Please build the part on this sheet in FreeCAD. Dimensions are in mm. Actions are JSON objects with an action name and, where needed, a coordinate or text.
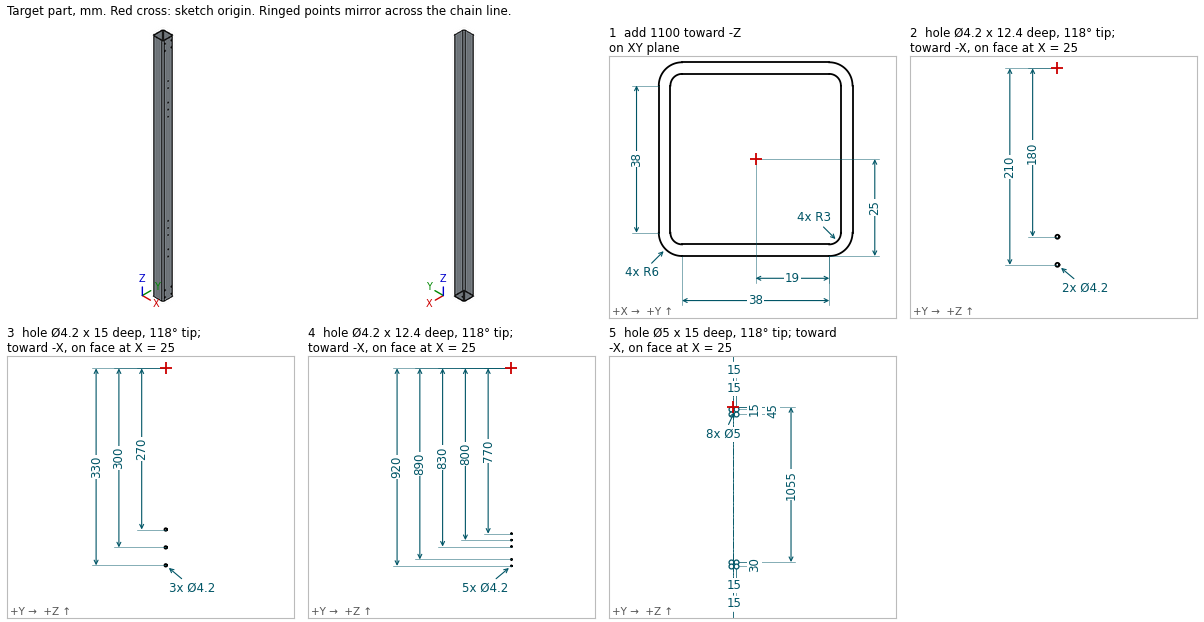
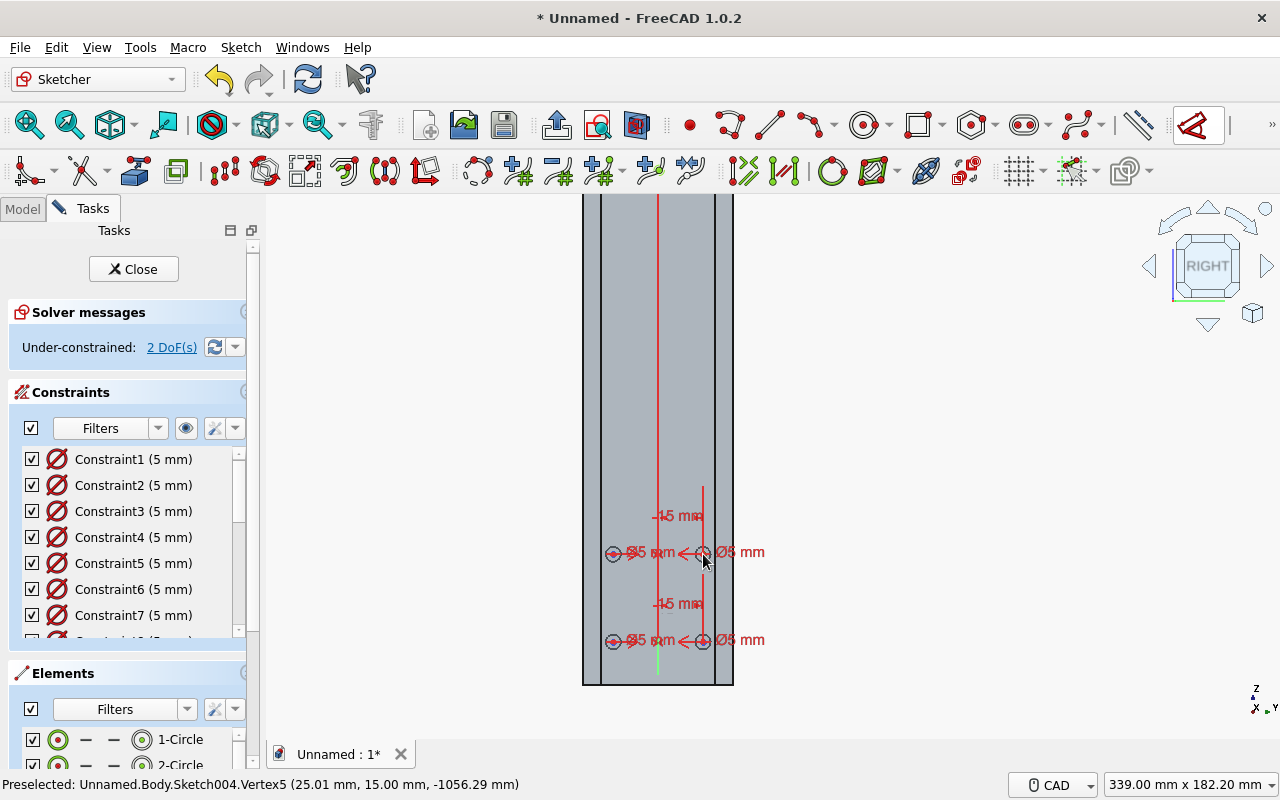
{"action": "left_click", "coordinate": [703, 642]}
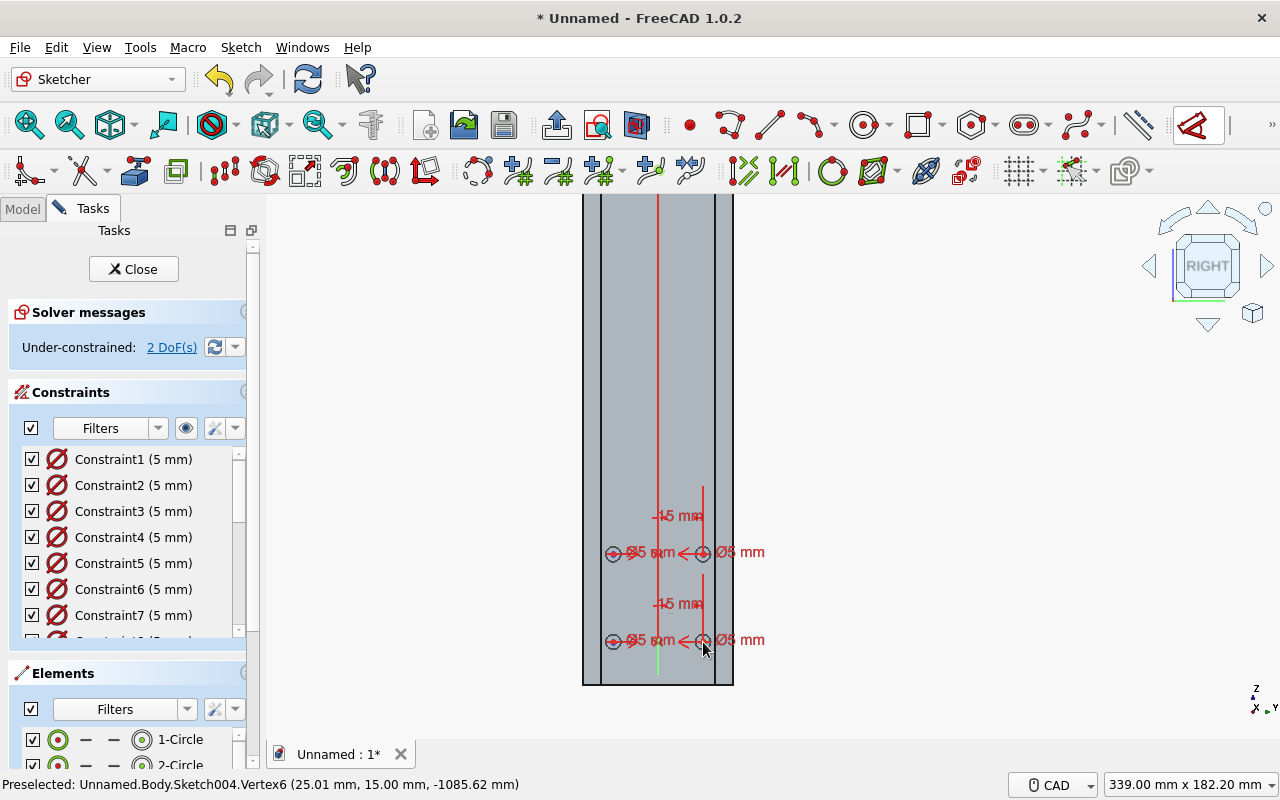
{"action": "left_click", "coordinate": [1218, 126]}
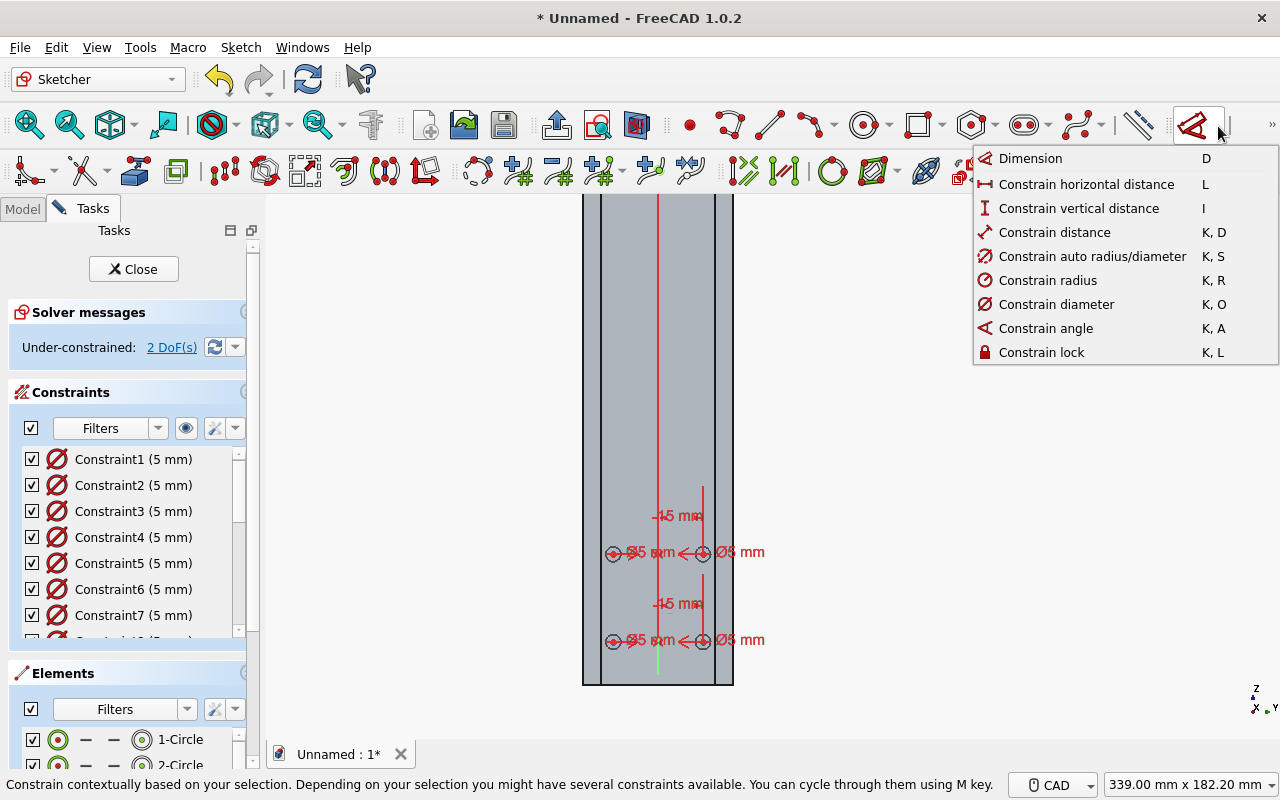
{"action": "left_click", "coordinate": [1126, 208]}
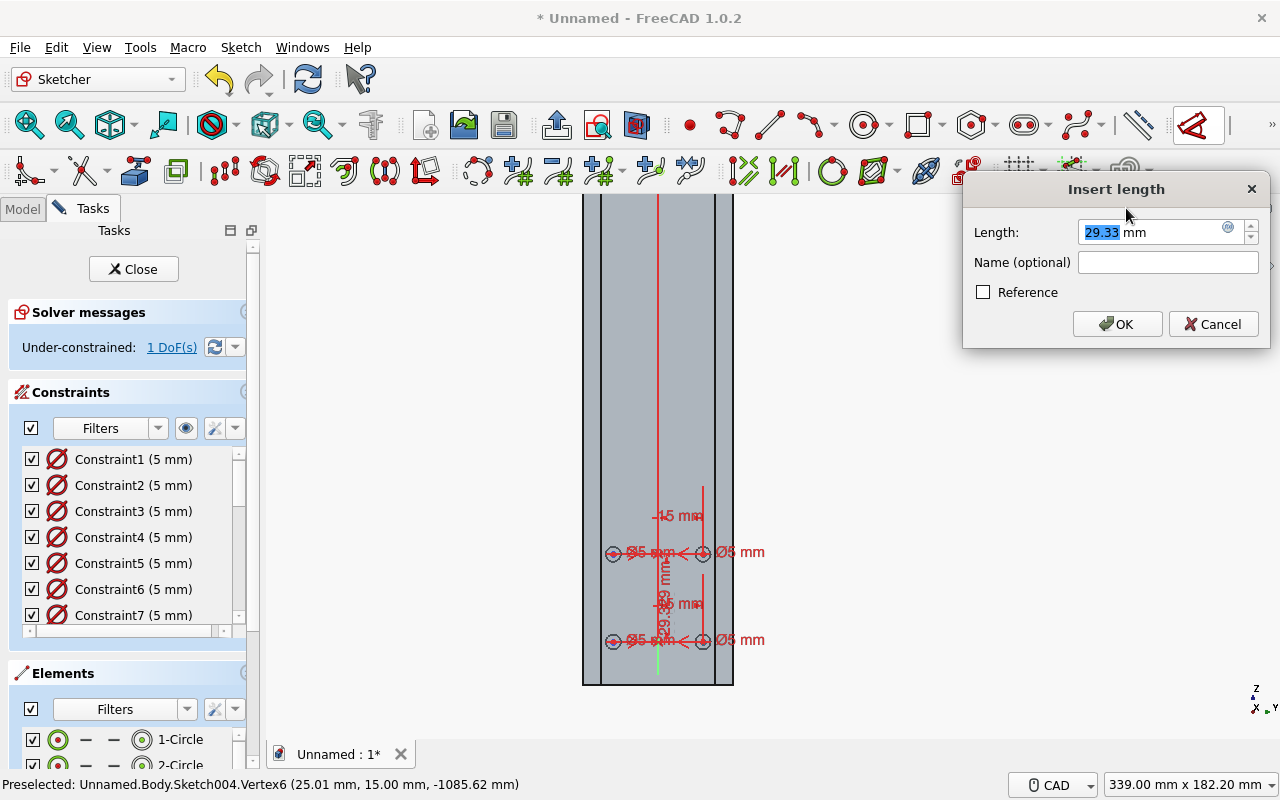
{"action": "type", "text": "30"}
{"action": "key", "text": "Return"}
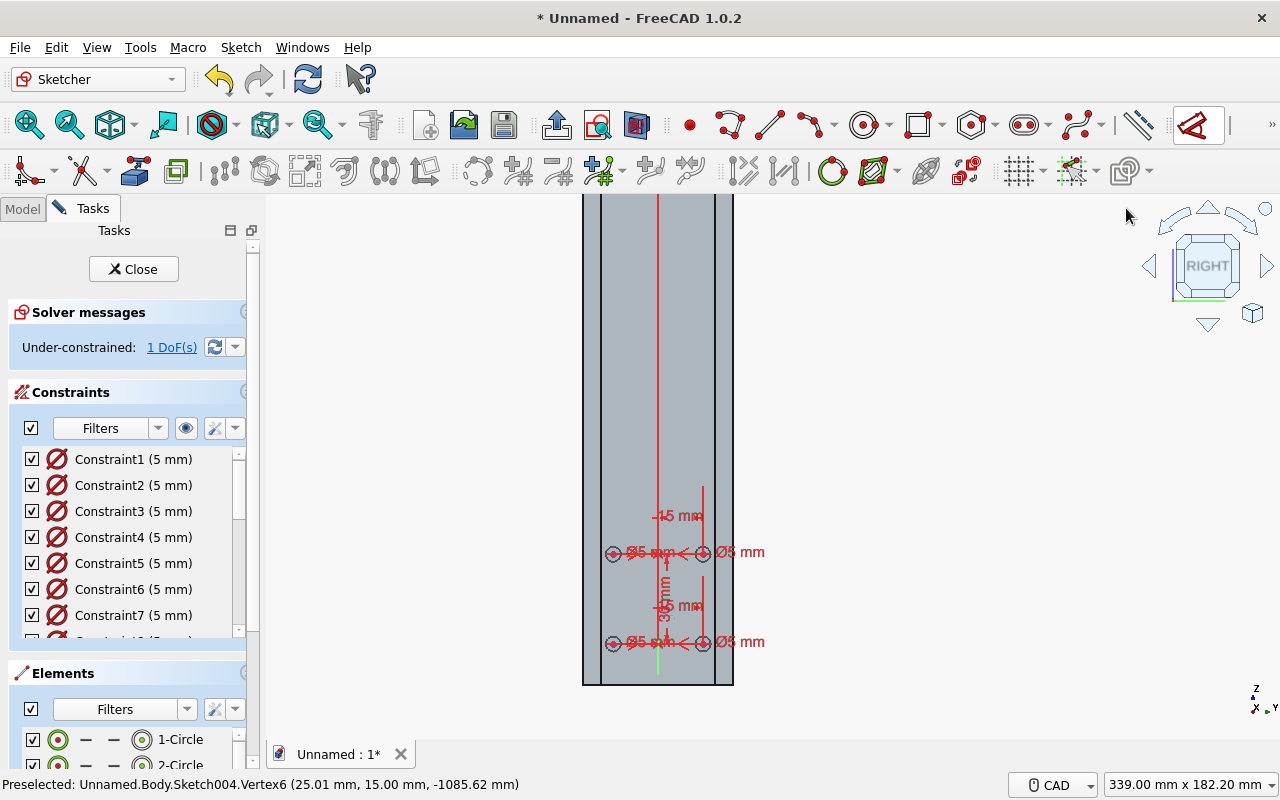
{"action": "scroll", "coordinate": [710, 647], "scroll_direction": "down", "scroll_amount": 11}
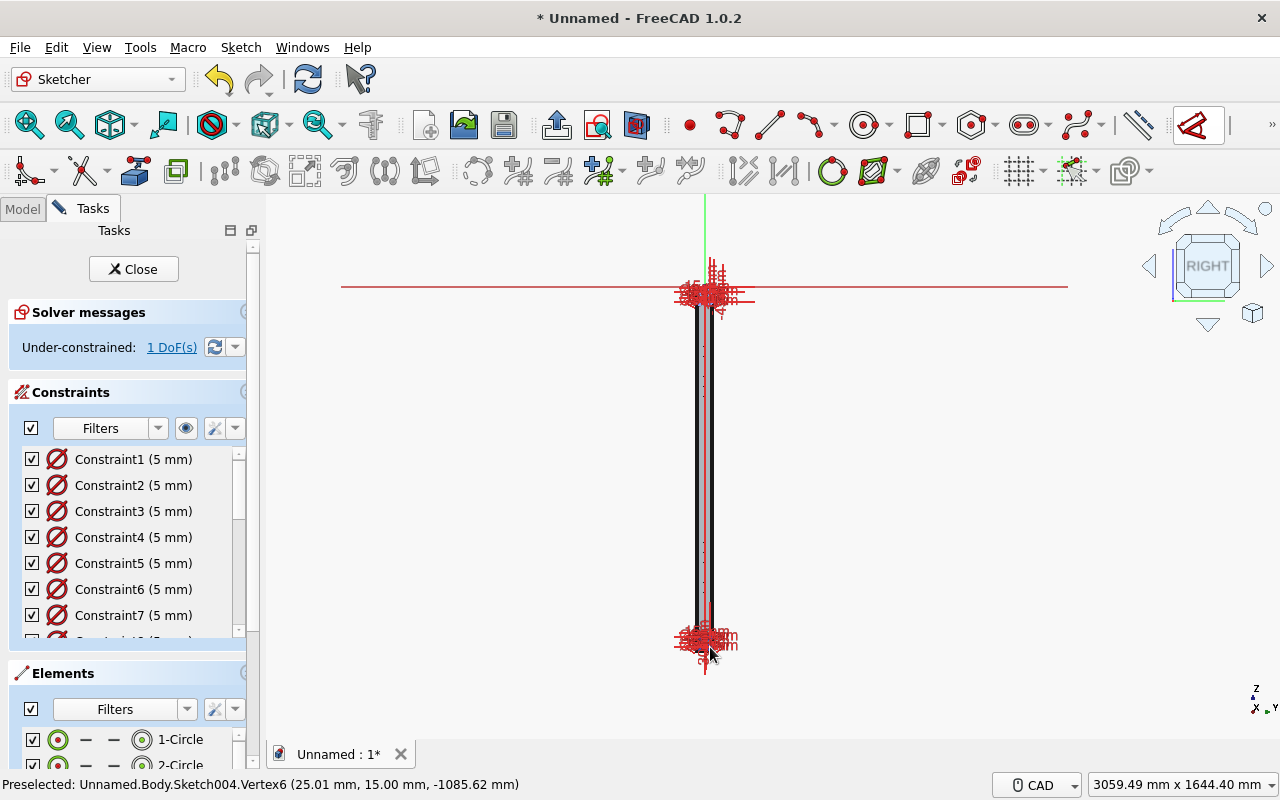
{"action": "scroll", "coordinate": [710, 637], "scroll_direction": "up", "scroll_amount": 2}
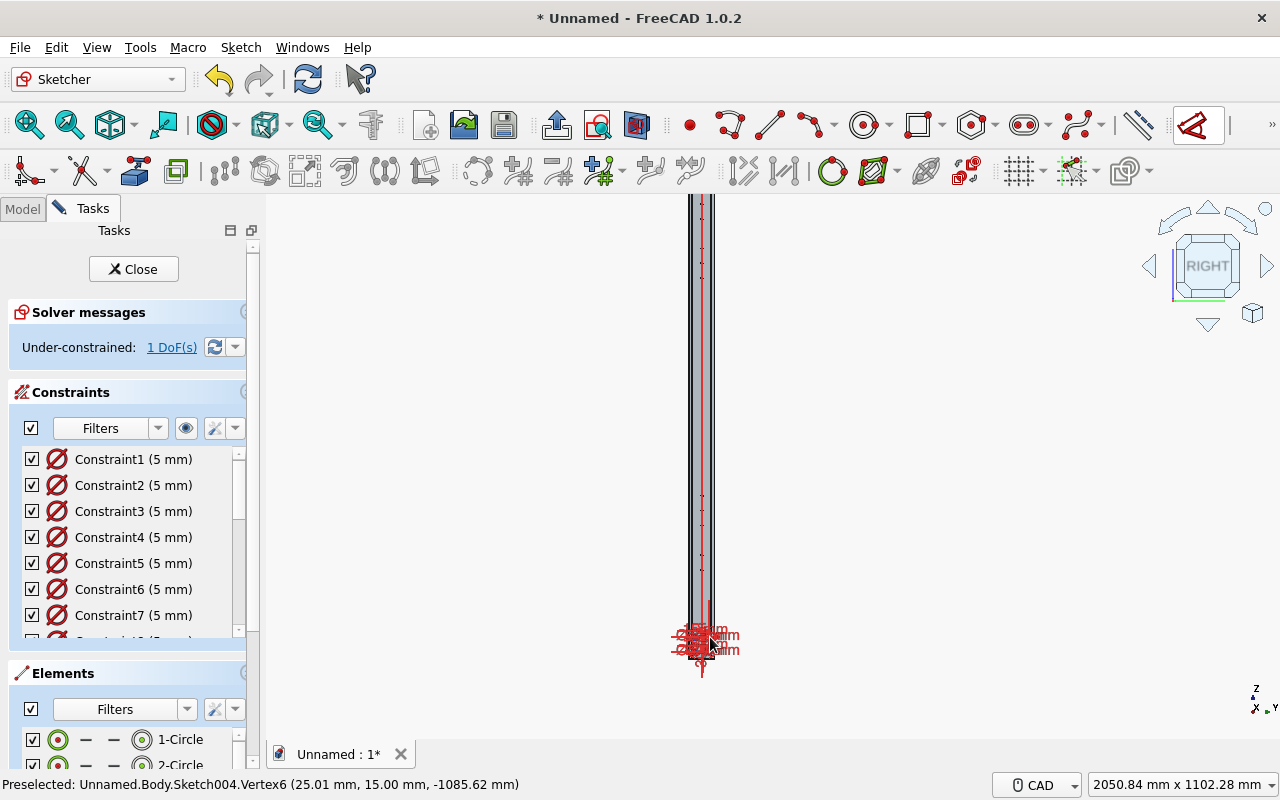
{"action": "left_click", "coordinate": [709, 637]}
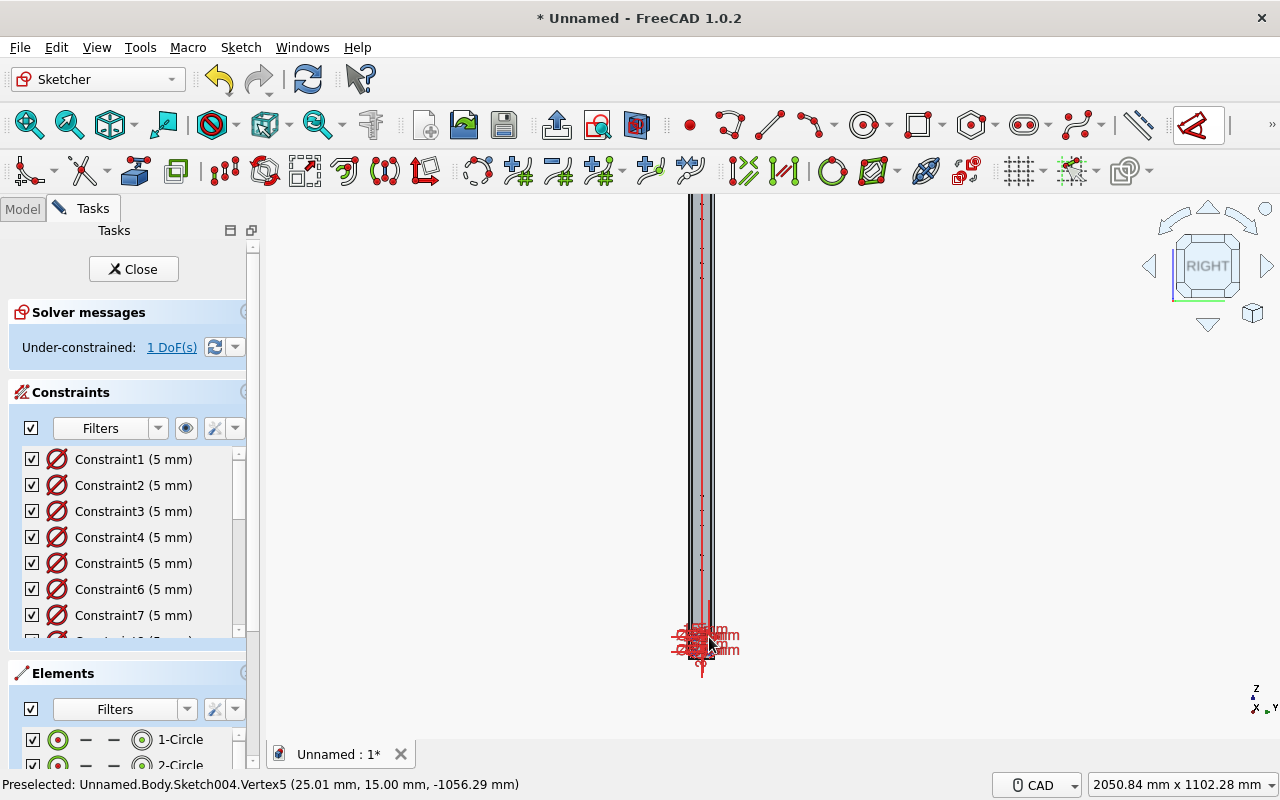
{"action": "left_click", "coordinate": [1218, 126]}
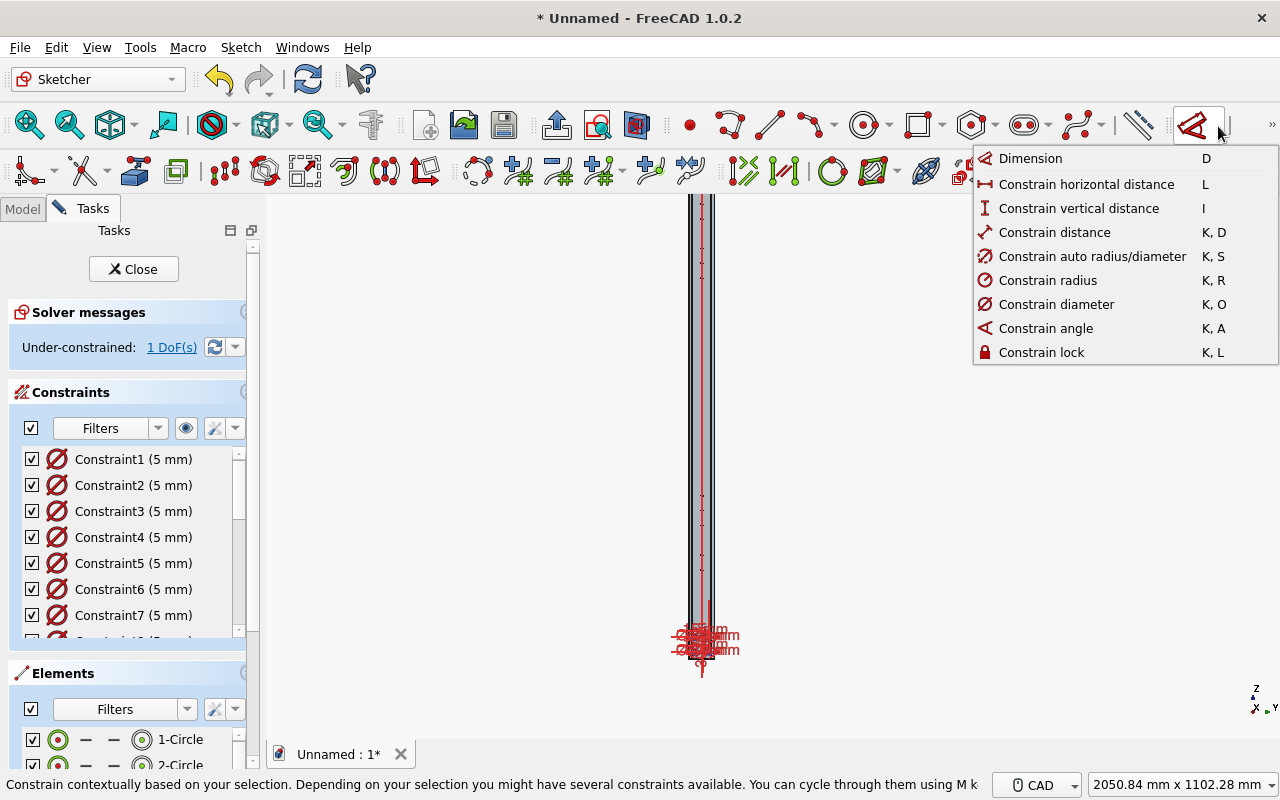
{"action": "left_click", "coordinate": [1126, 208]}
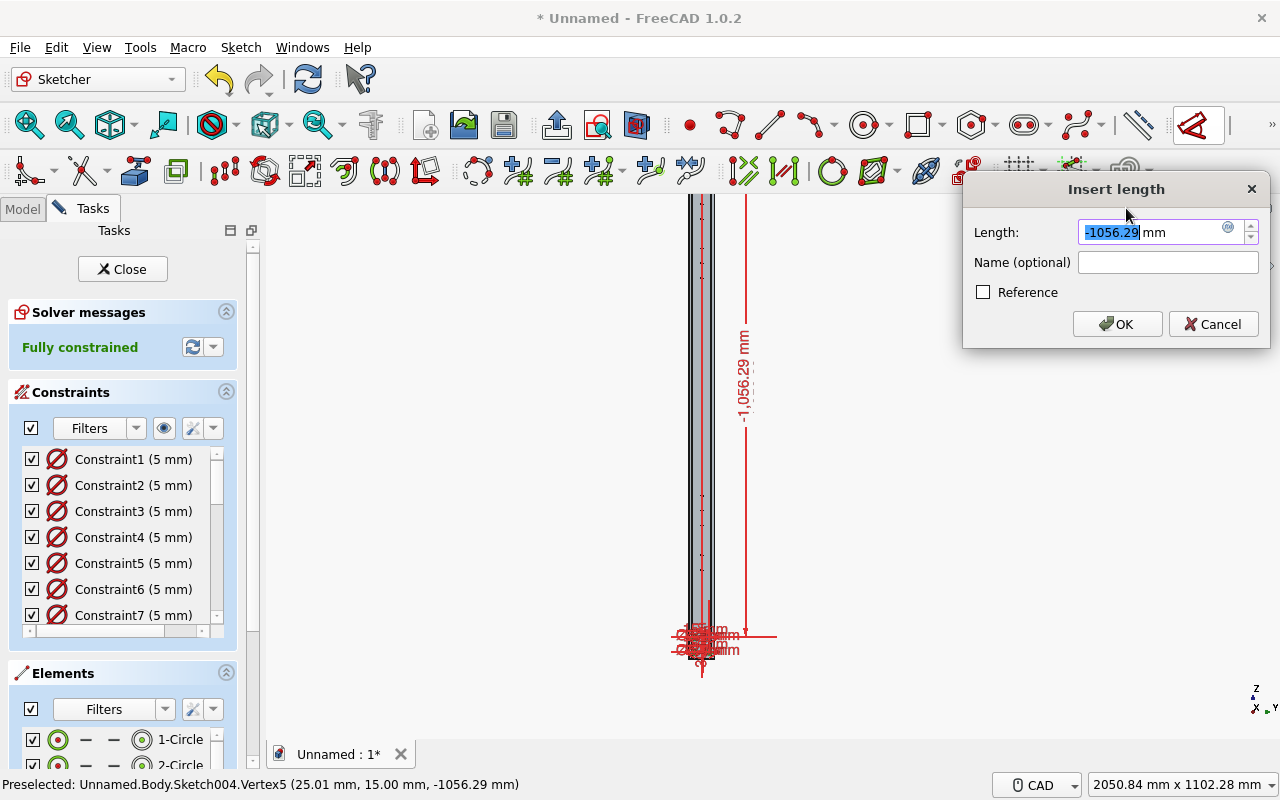
{"action": "type", "text": "-1055"}
{"action": "key", "text": "Return"}